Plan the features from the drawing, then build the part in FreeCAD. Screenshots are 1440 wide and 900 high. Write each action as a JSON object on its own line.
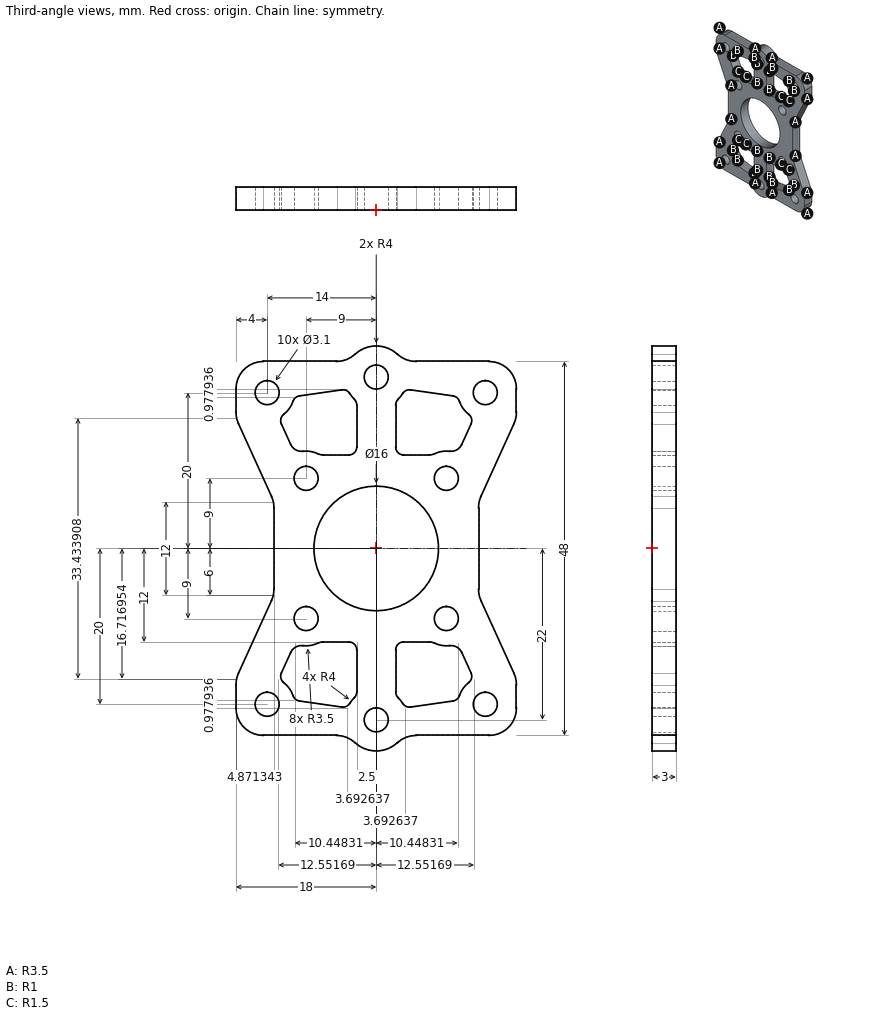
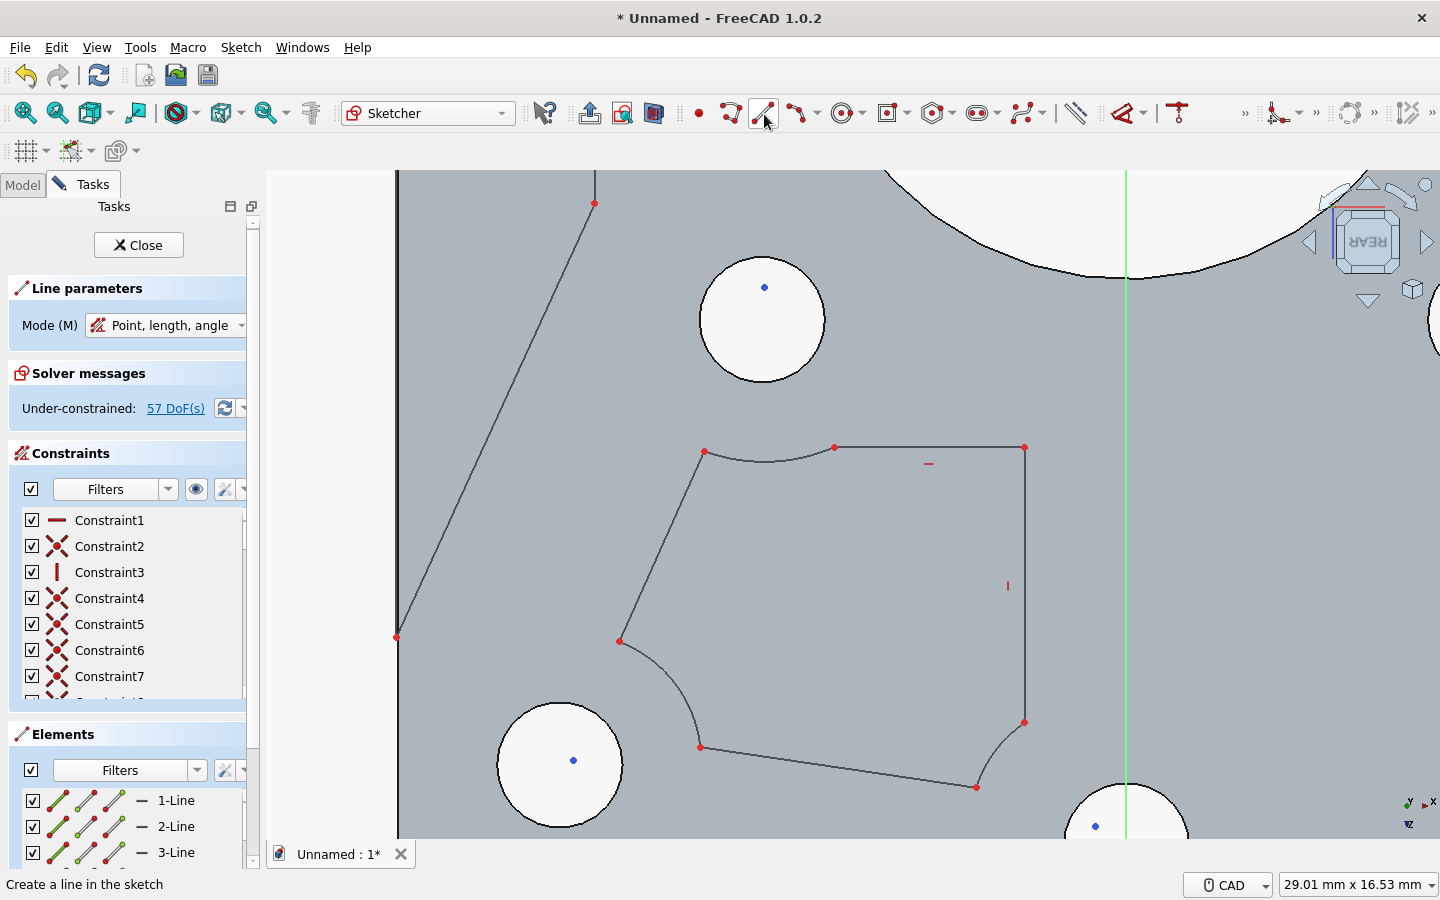
{"action": "scroll", "coordinate": [673, 684], "scroll_direction": "down", "scroll_amount": 7}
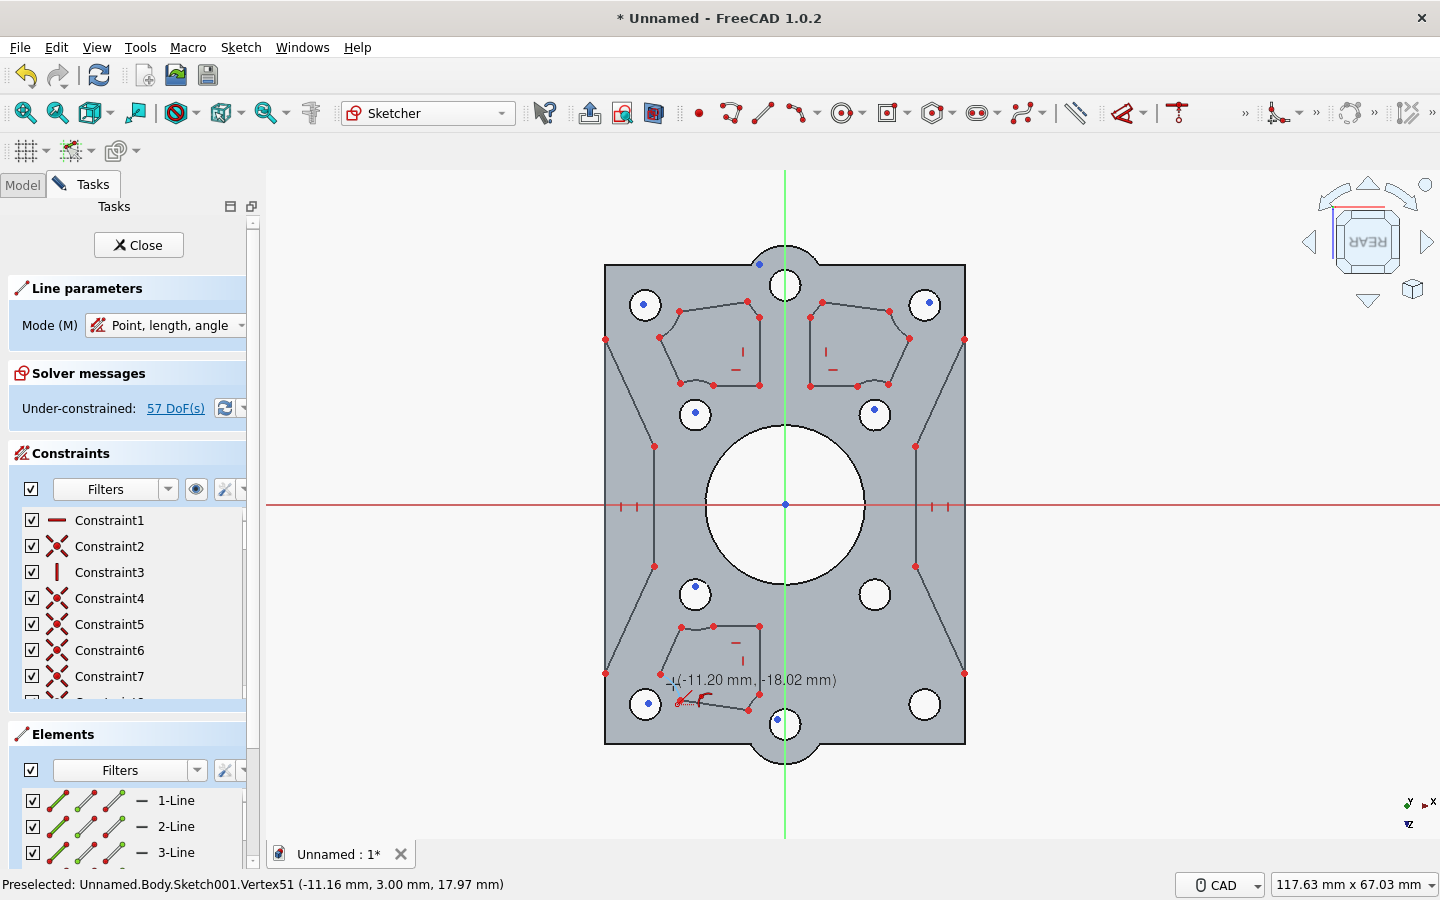
{"action": "left_click", "coordinate": [822, 709]}
{"action": "left_click", "coordinate": [890, 699]}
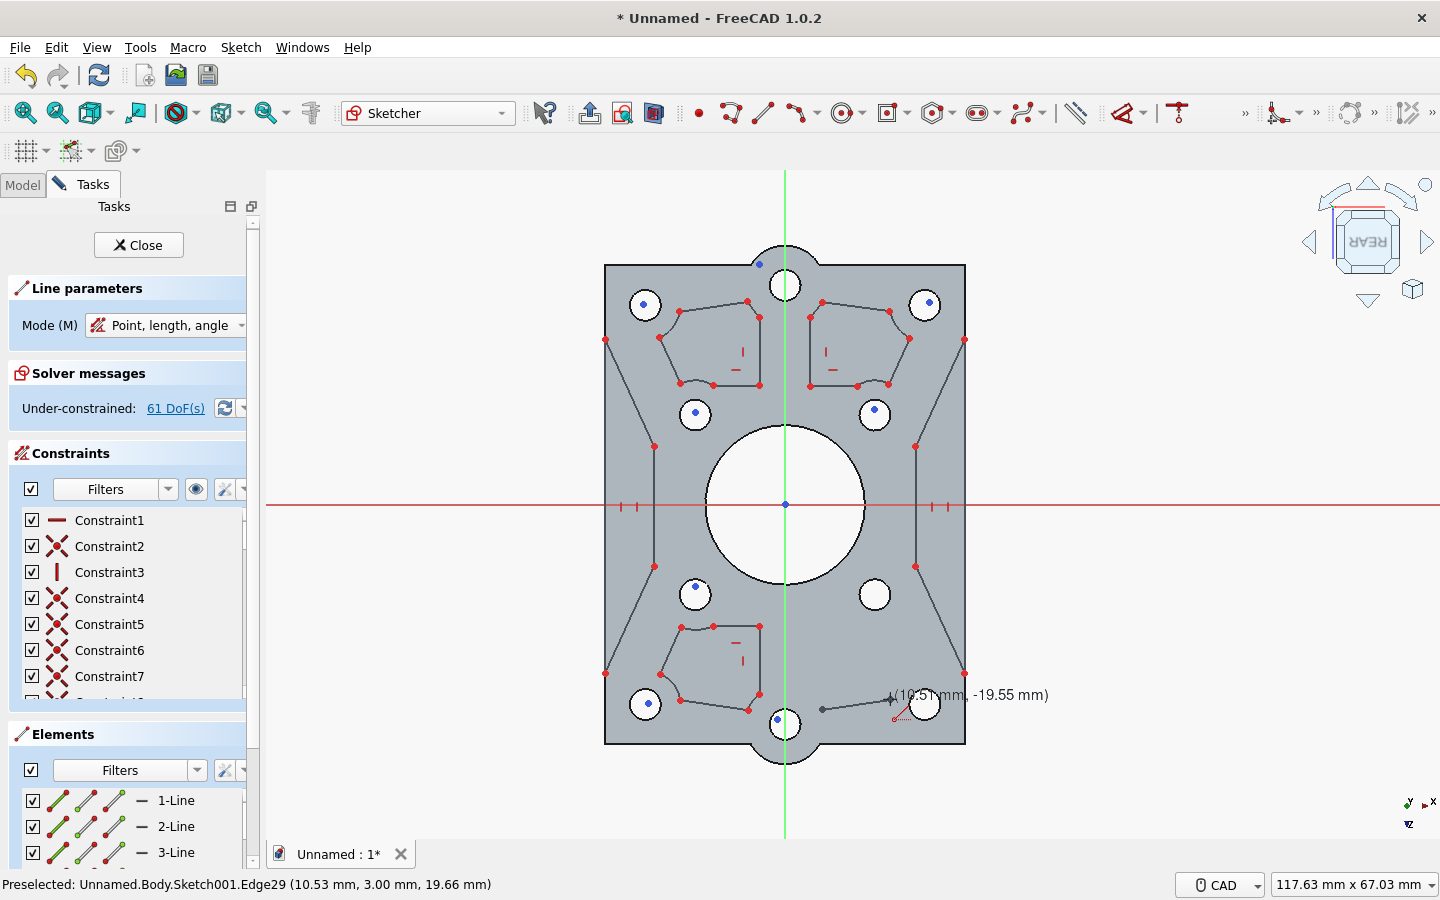
{"action": "left_click", "coordinate": [910, 673]}
{"action": "left_click", "coordinate": [889, 627]}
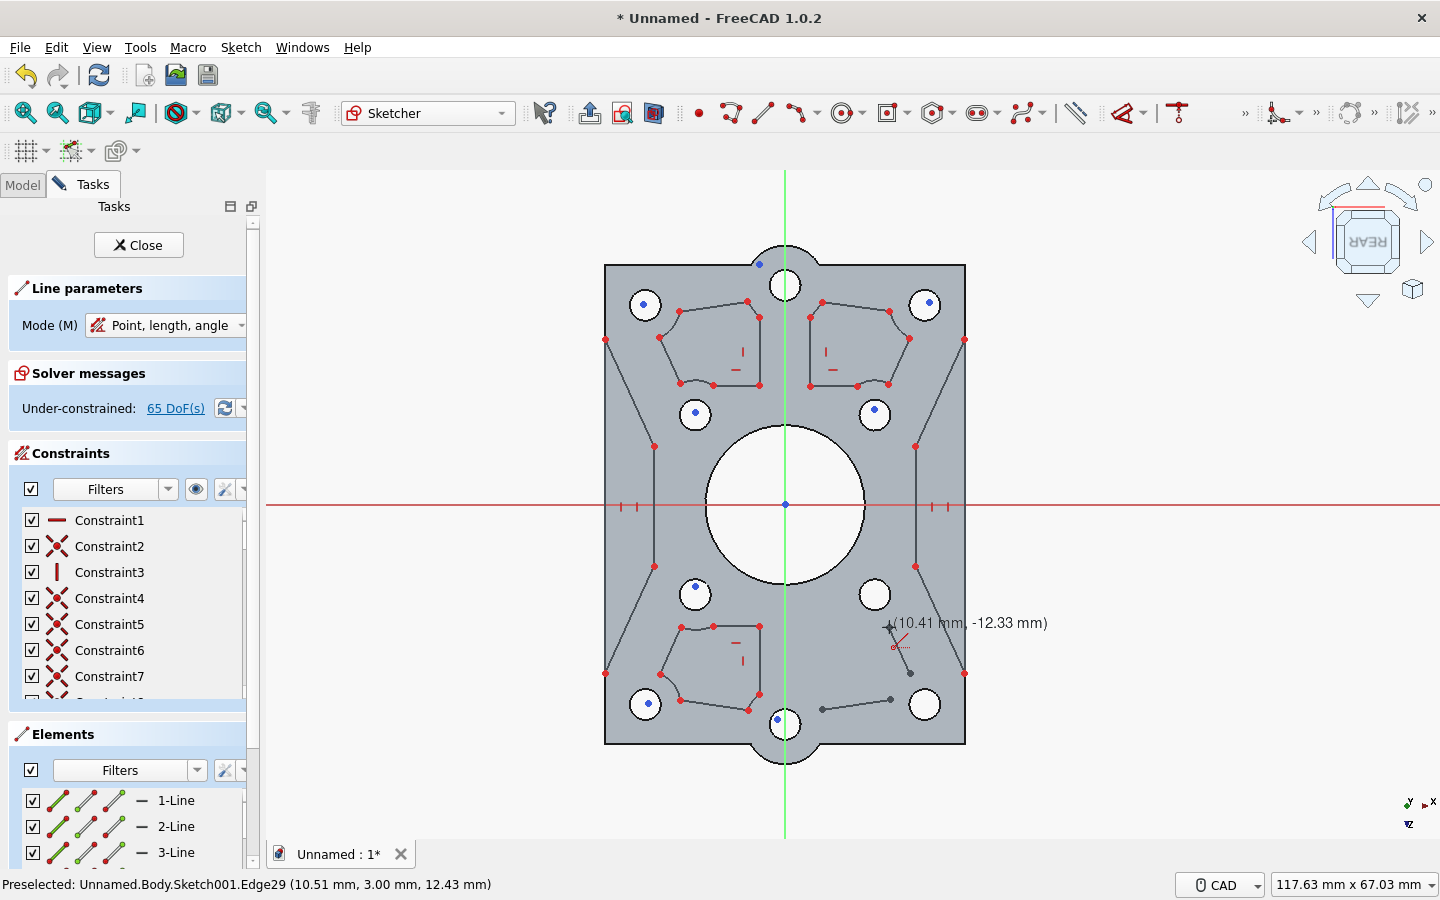
{"action": "key", "text": "g m"}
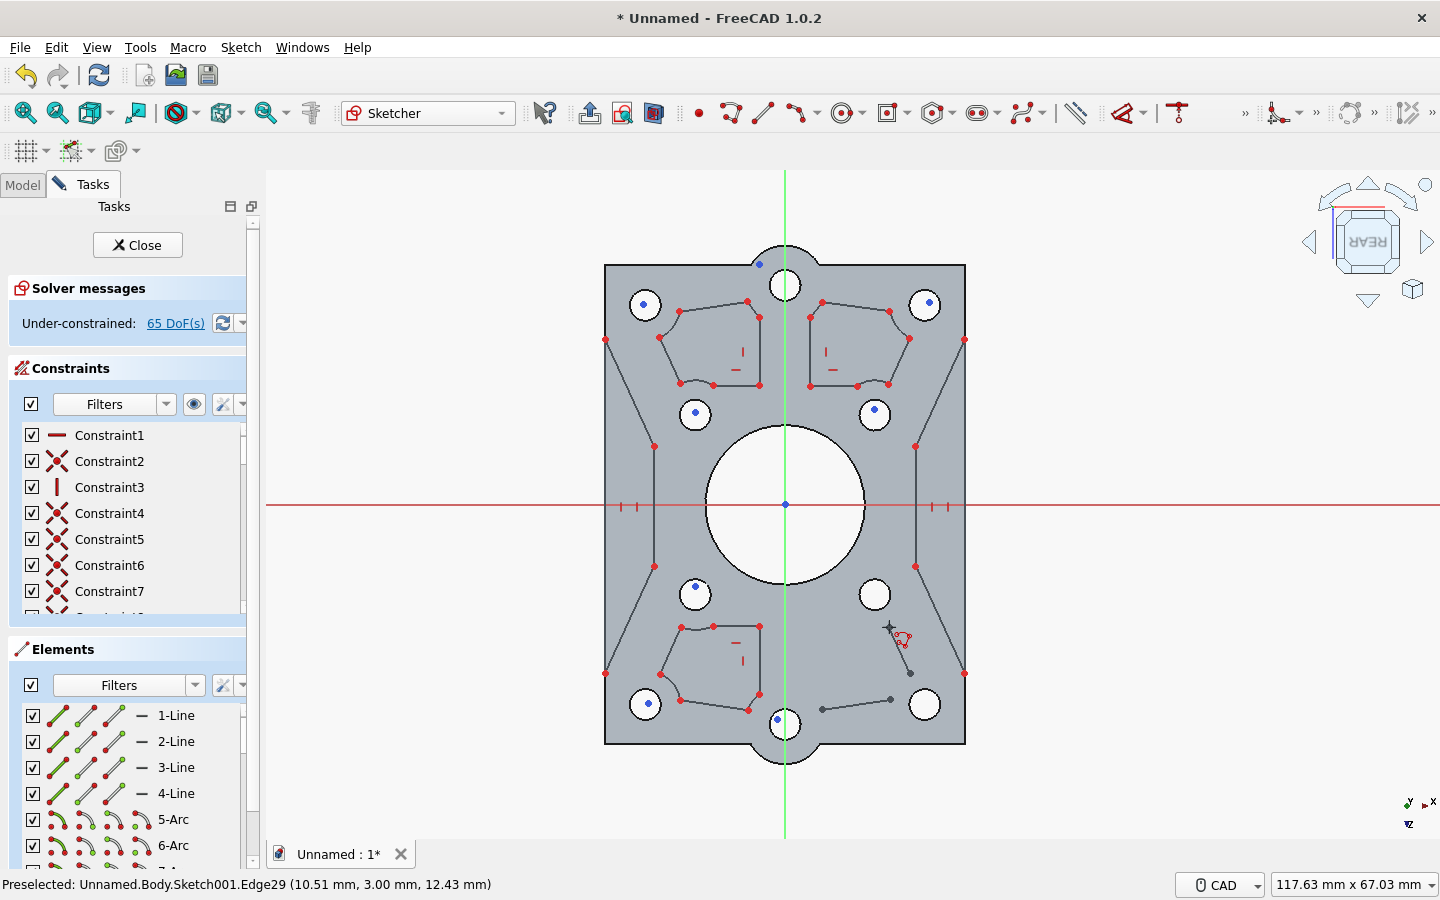
{"action": "left_click", "coordinate": [857, 625]}
{"action": "left_click", "coordinate": [810, 625]}
{"action": "left_click", "coordinate": [810, 693]}
{"action": "right_click", "coordinate": [810, 693]}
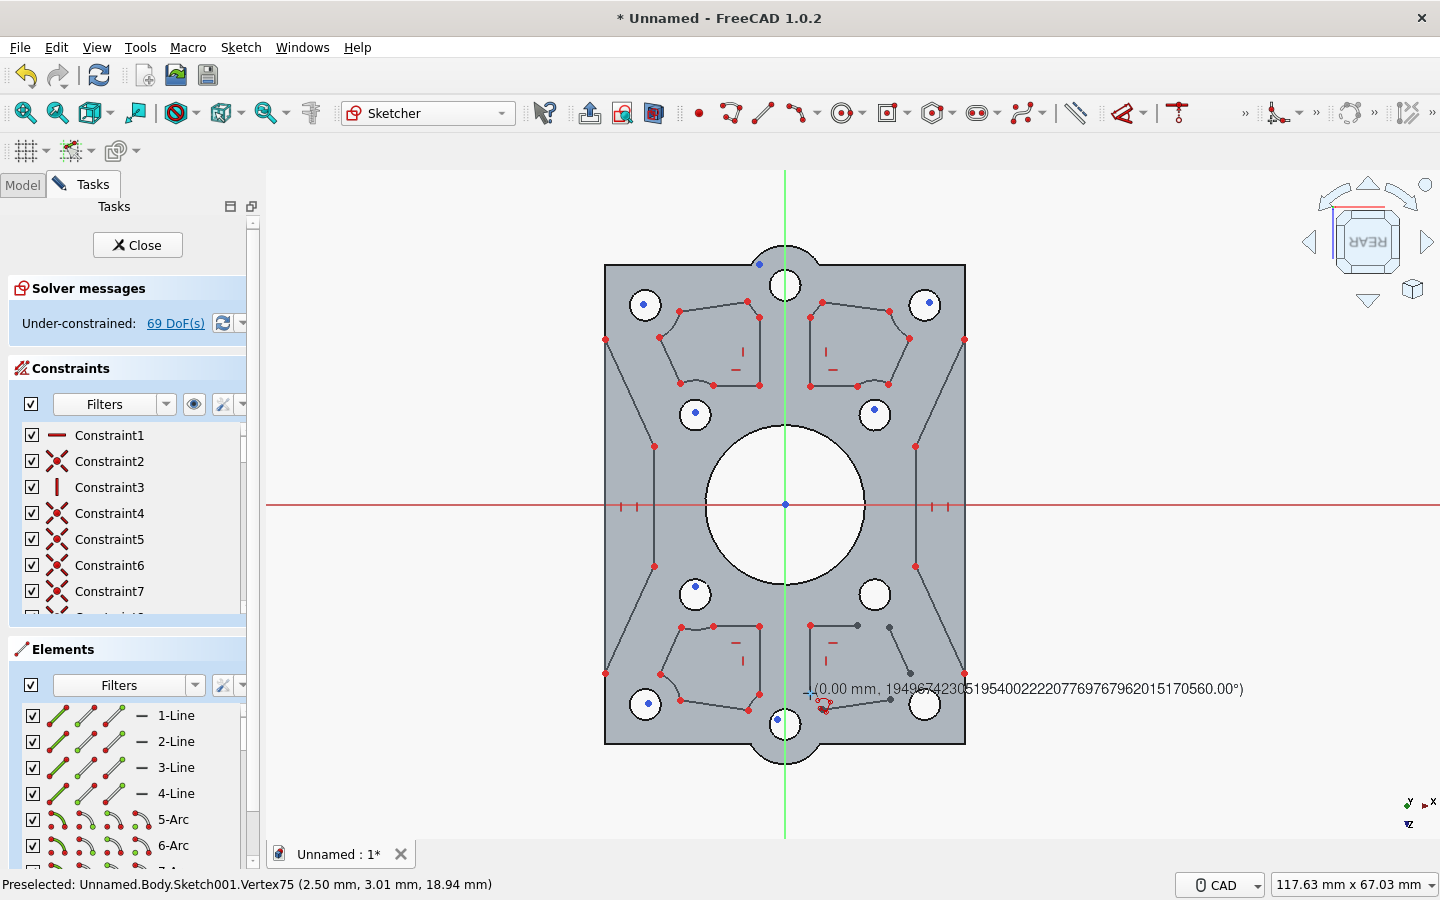
{"action": "left_click", "coordinate": [796, 114]}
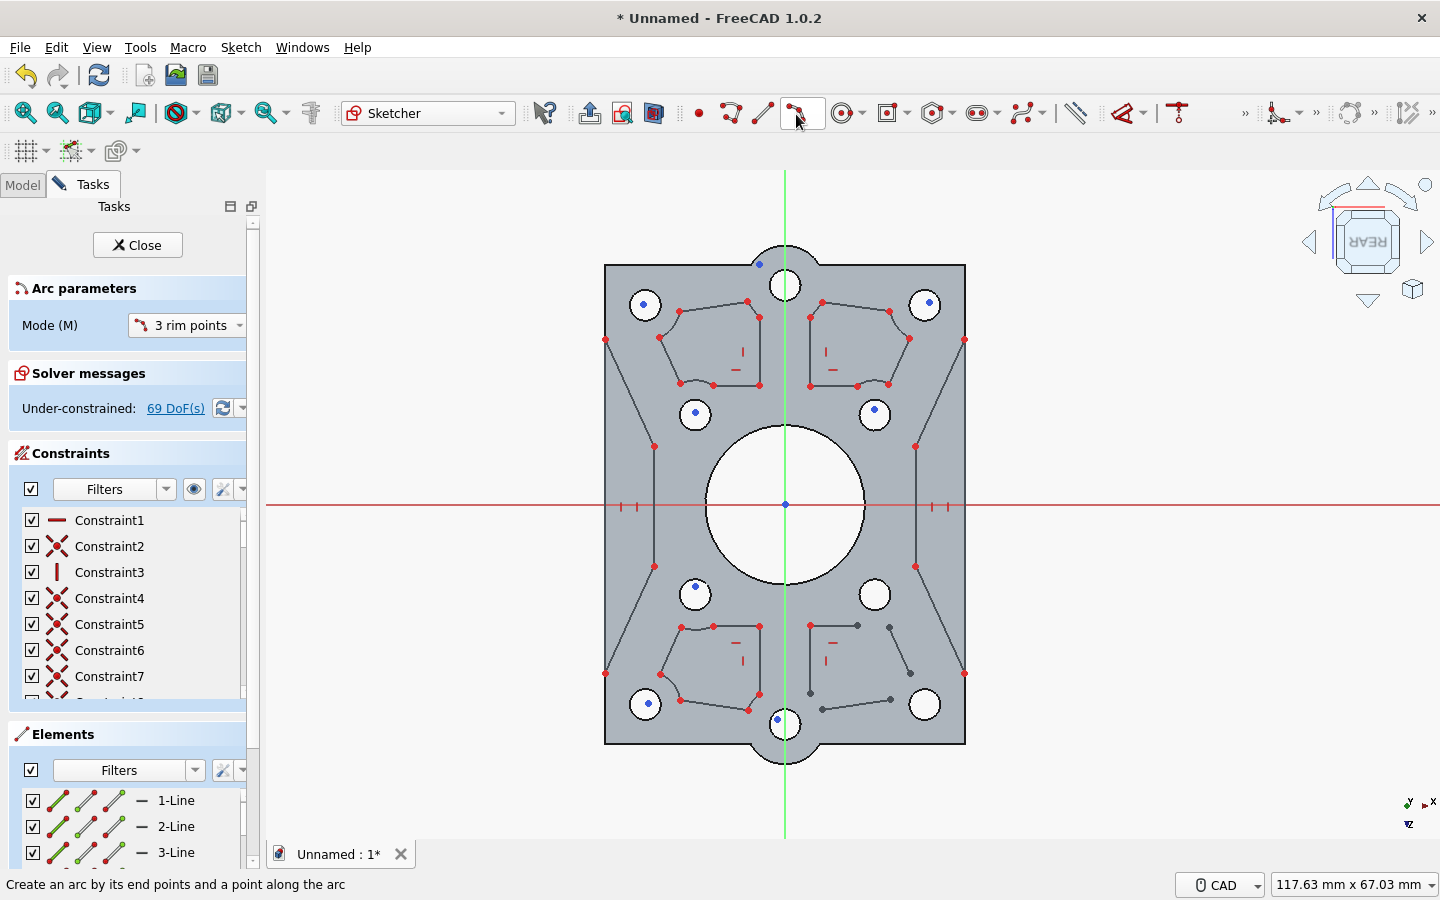
{"action": "left_click", "coordinate": [890, 700]}
{"action": "left_click", "coordinate": [910, 674]}